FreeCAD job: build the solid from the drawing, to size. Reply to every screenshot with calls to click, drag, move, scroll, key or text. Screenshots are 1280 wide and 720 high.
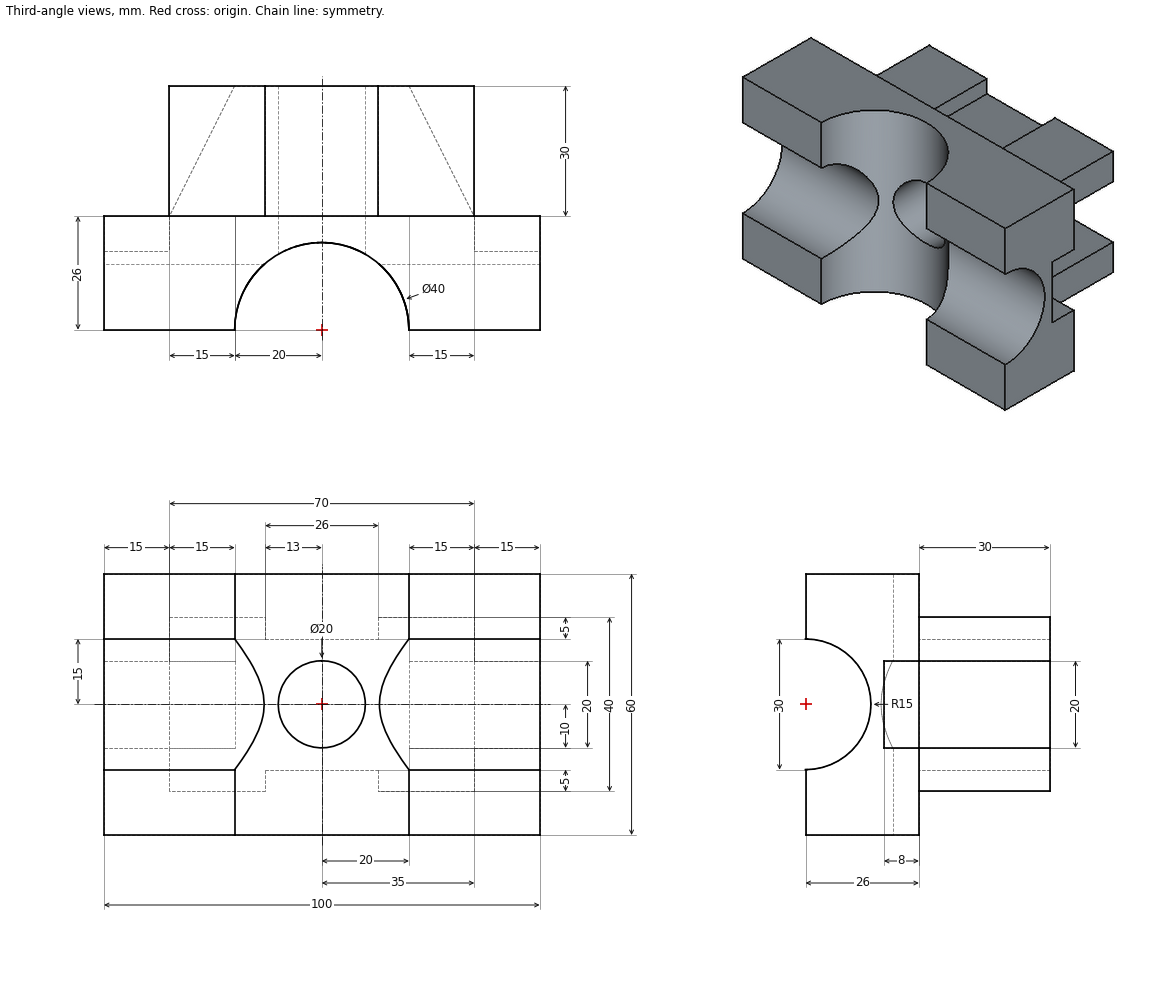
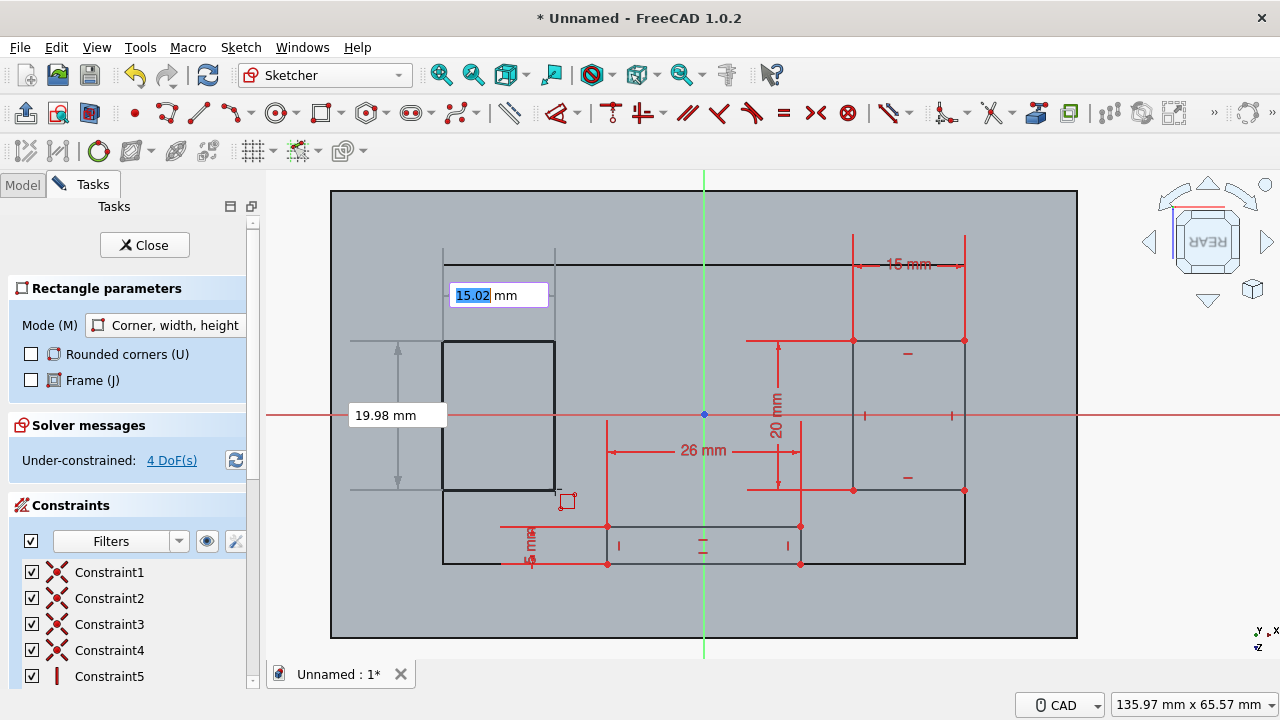
text(15)
key(Tab)
text(20)
key(Return)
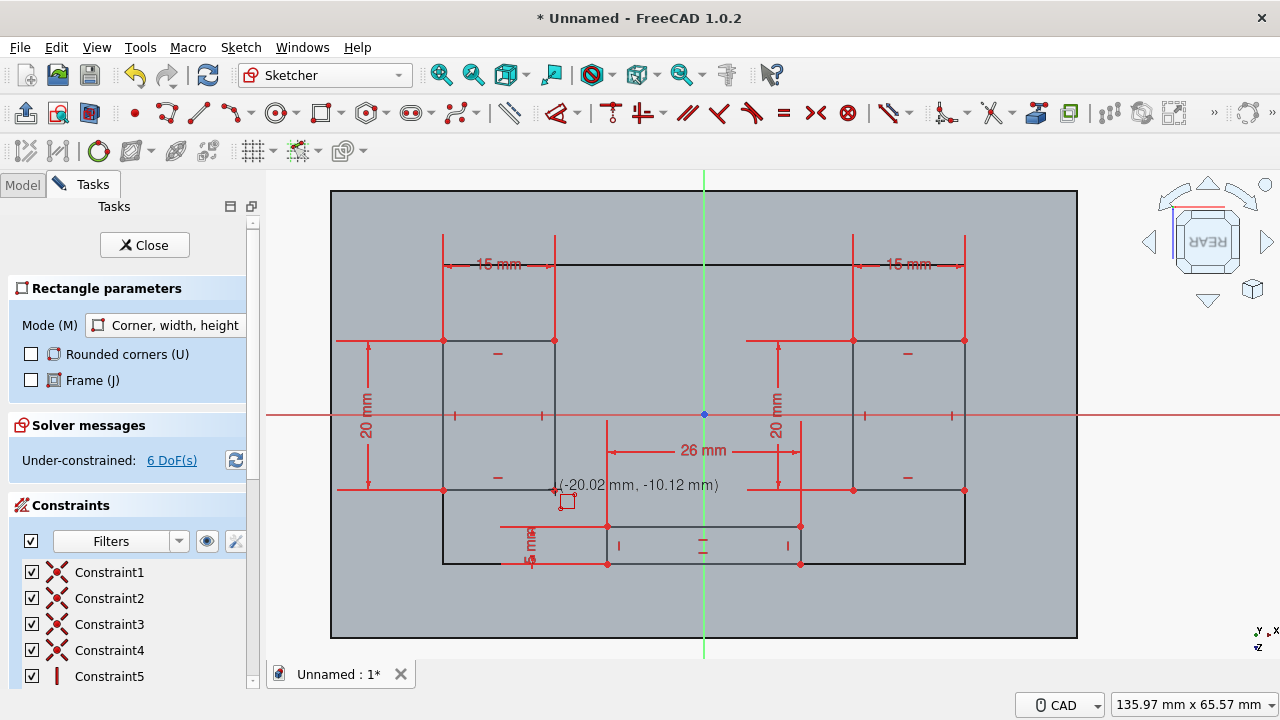
click(607, 265)
move(801, 303)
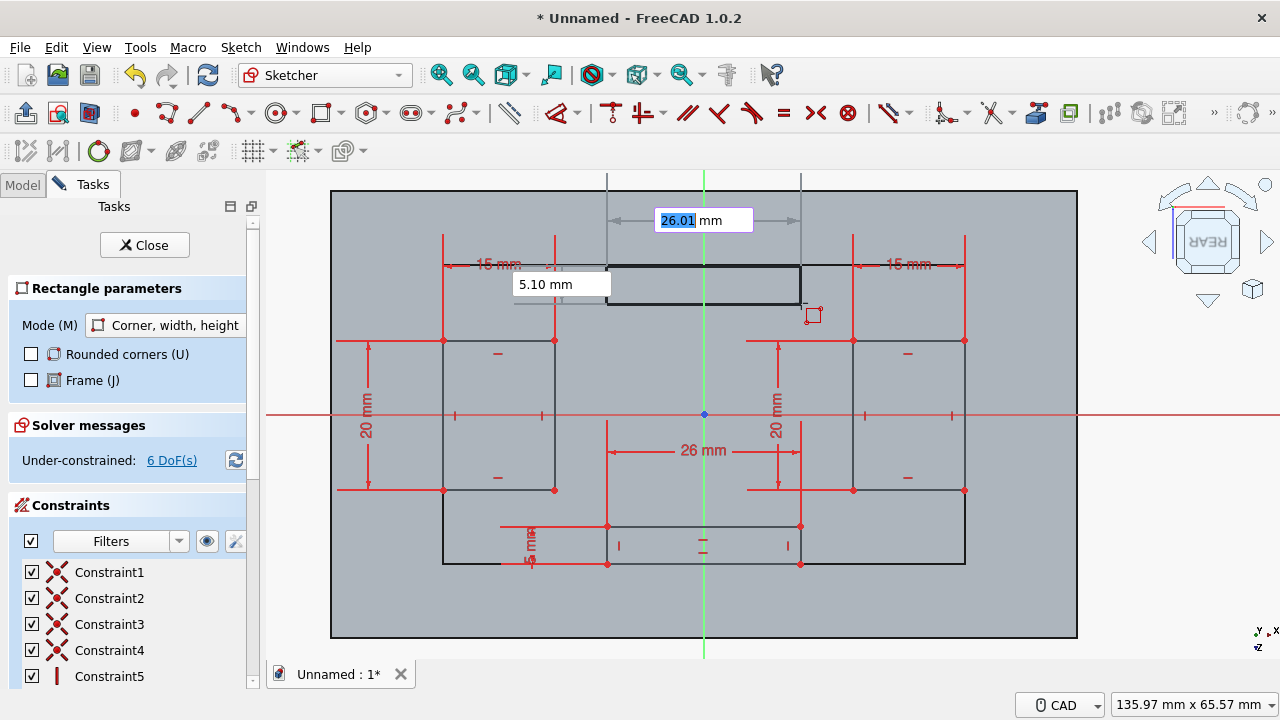
text(26)
key(Tab)
text(5)
key(Return)
key(Escape)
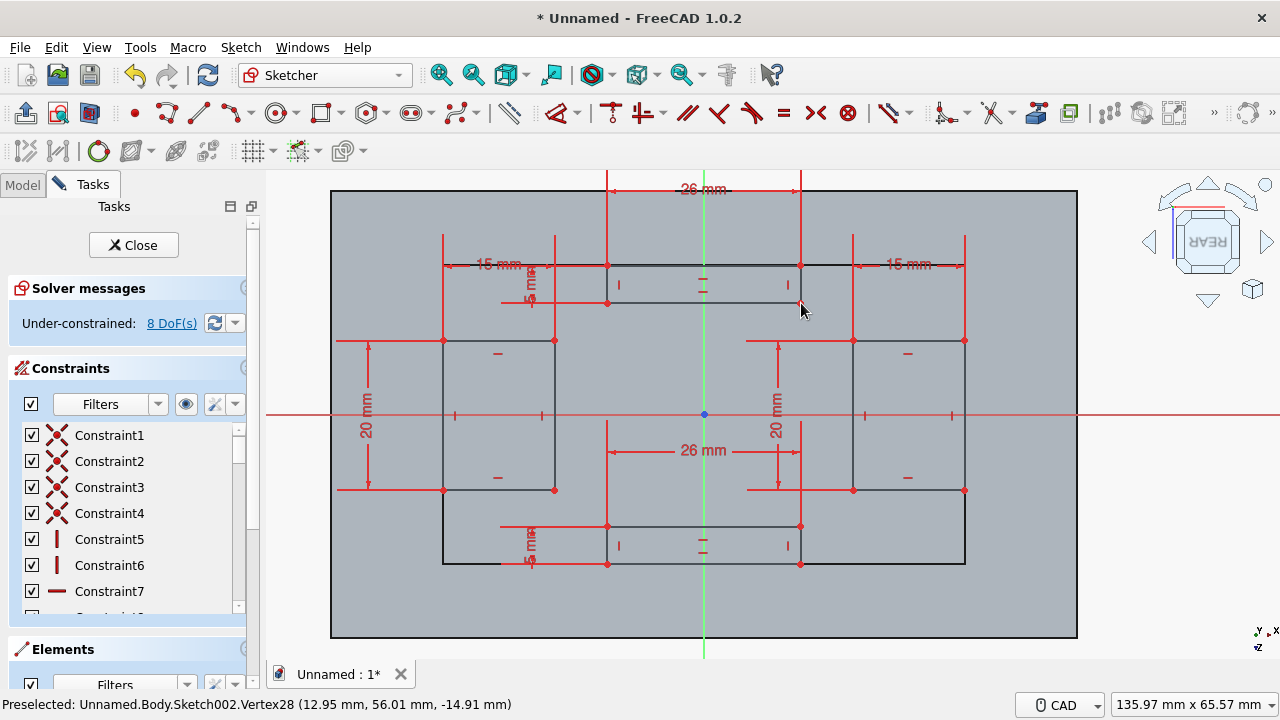
click(965, 341)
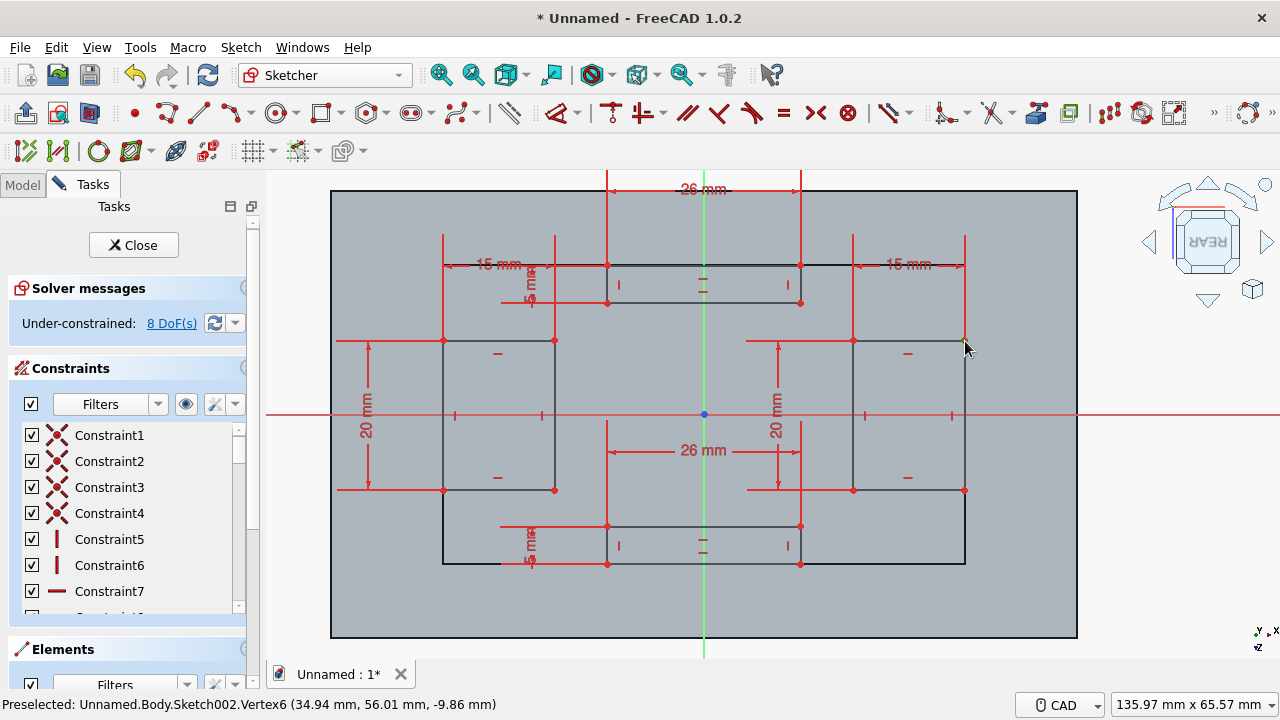
click(443, 341)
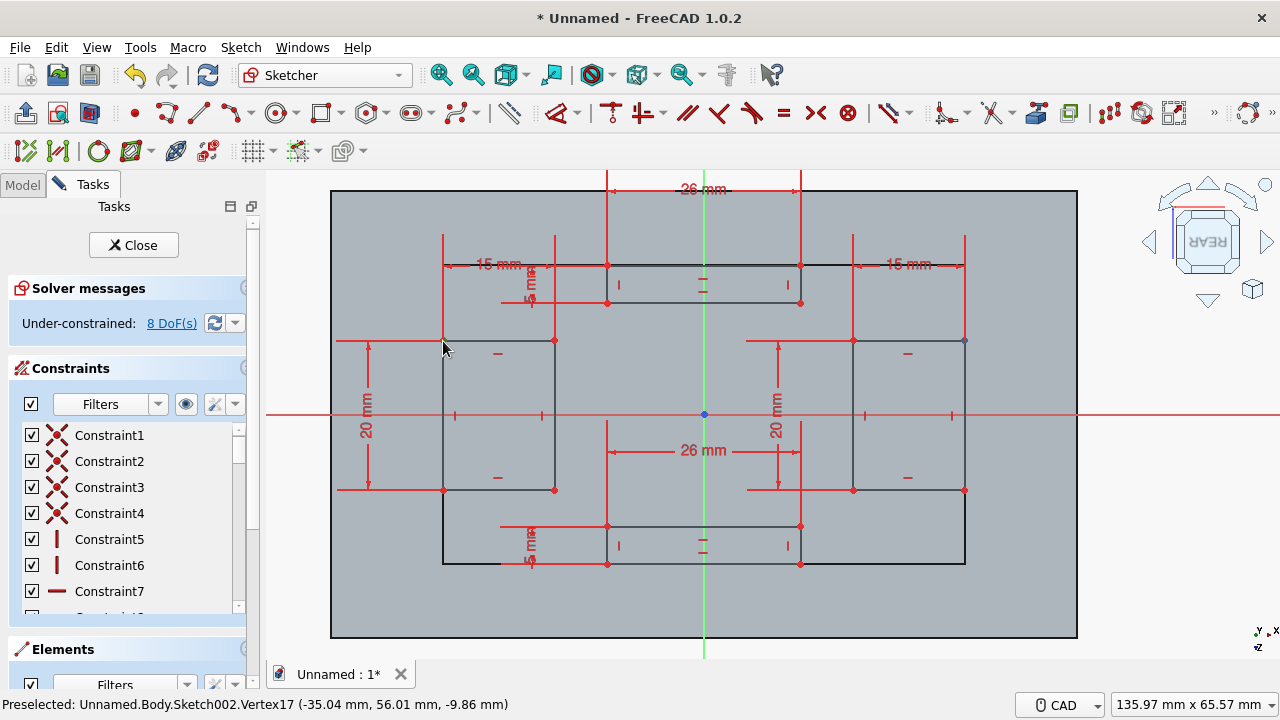
click(704, 600)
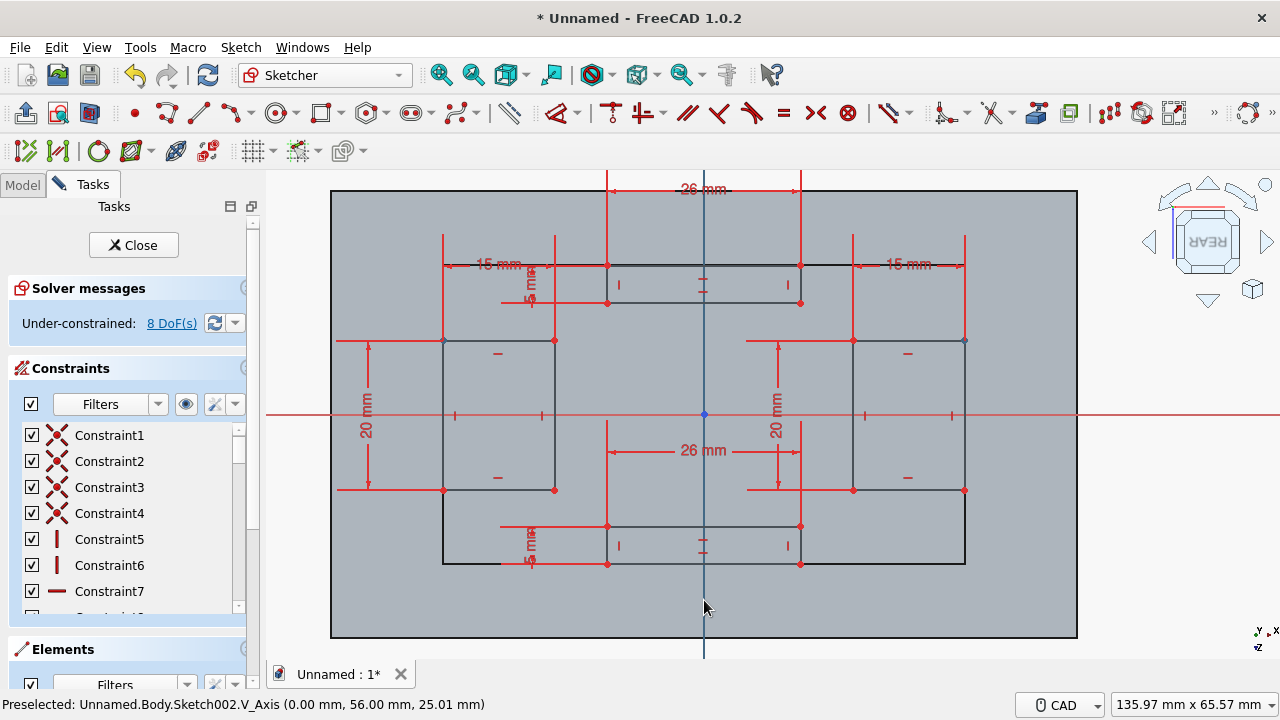
key(s)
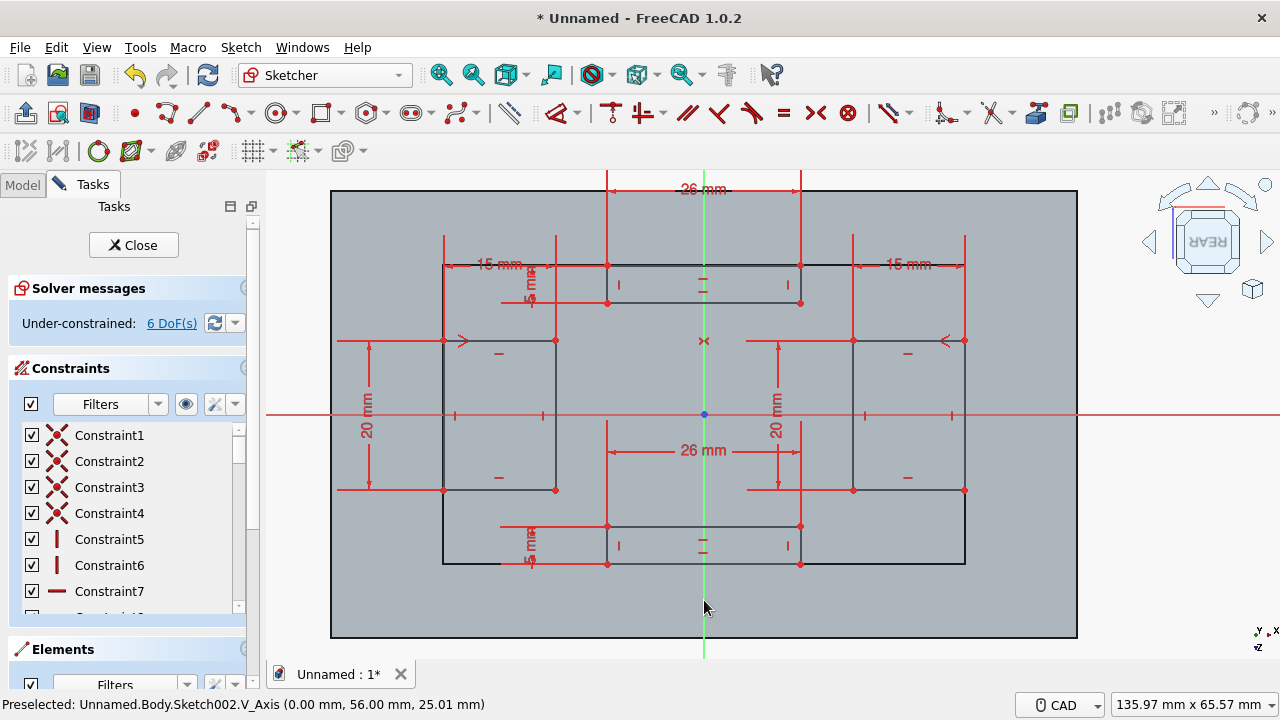
click(607, 564)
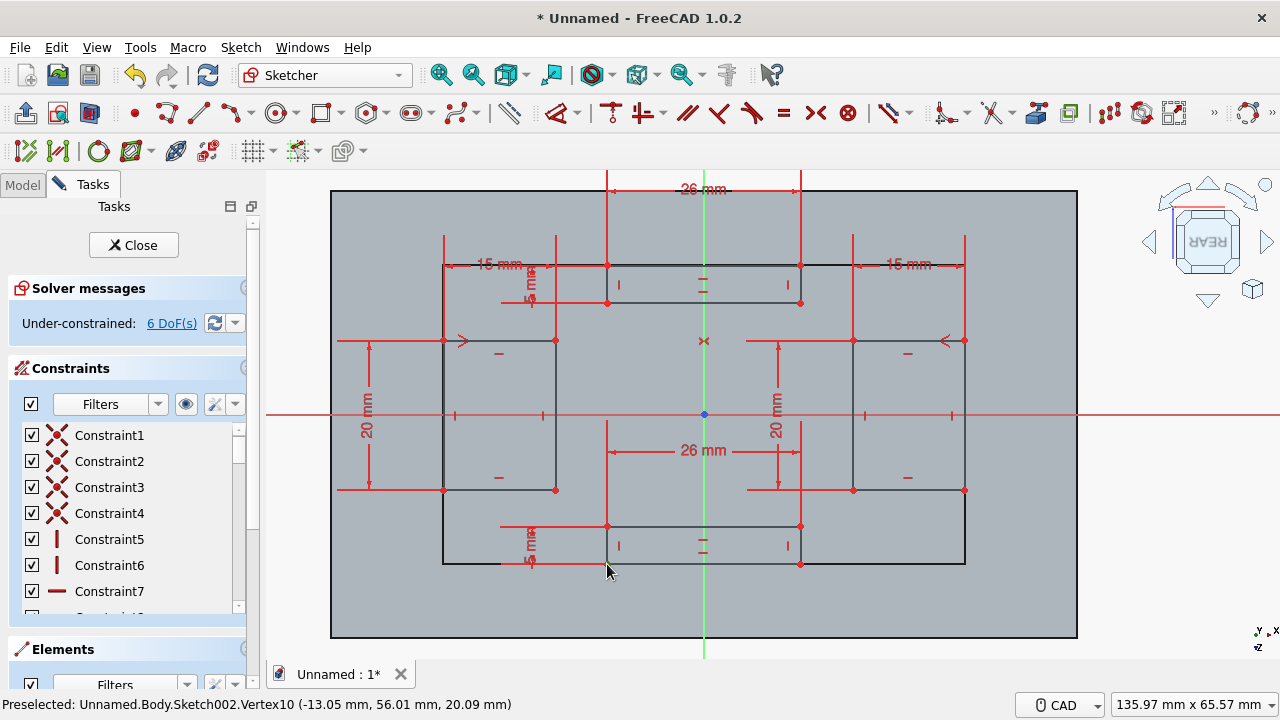
click(607, 266)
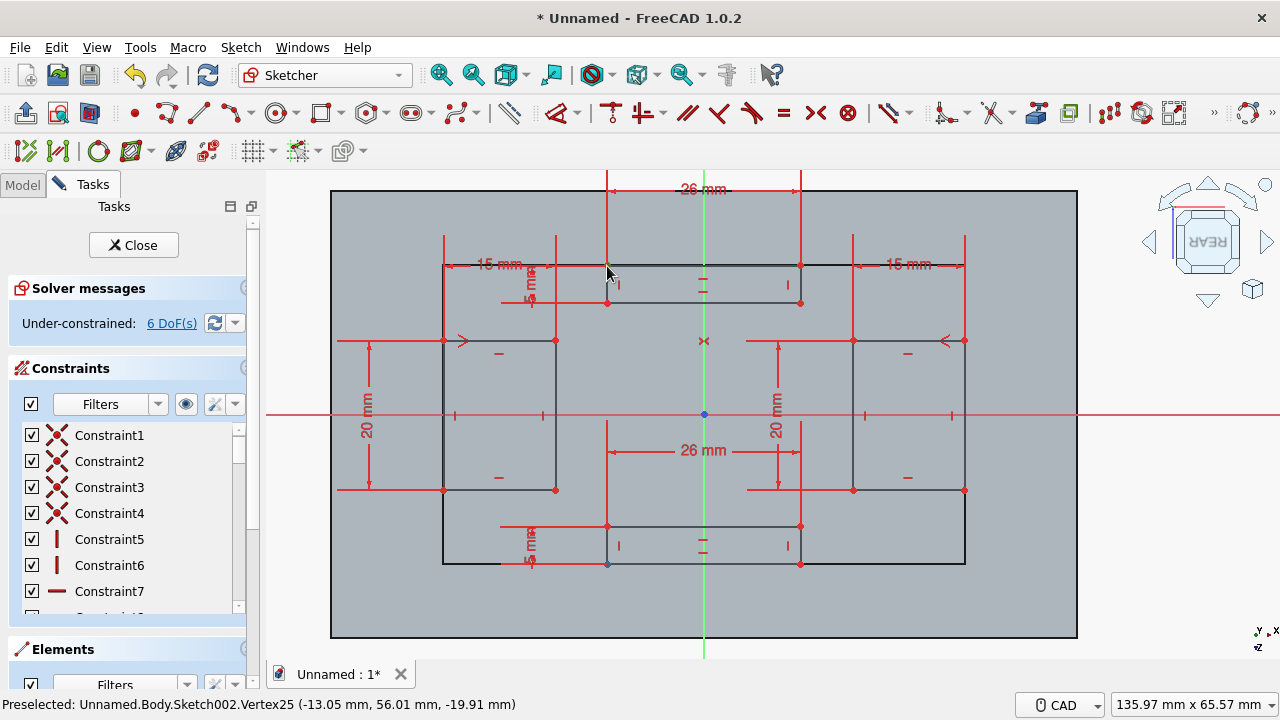
click(353, 414)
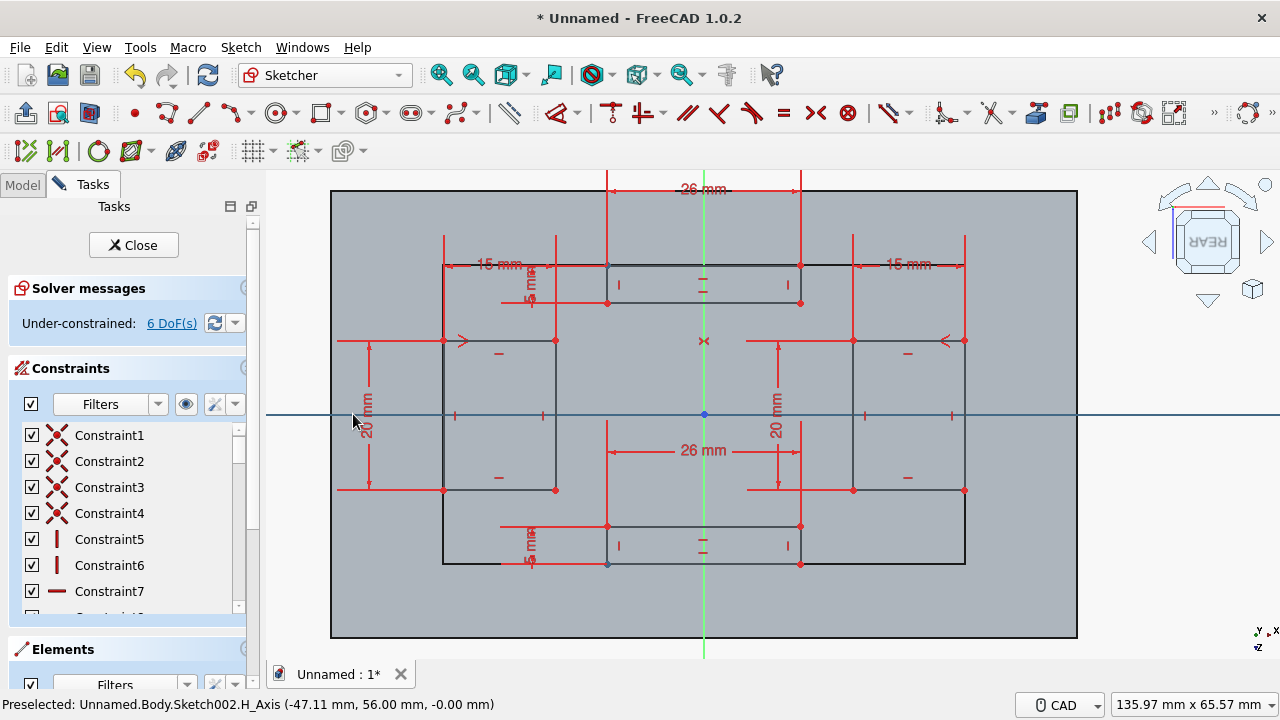
click(816, 114)